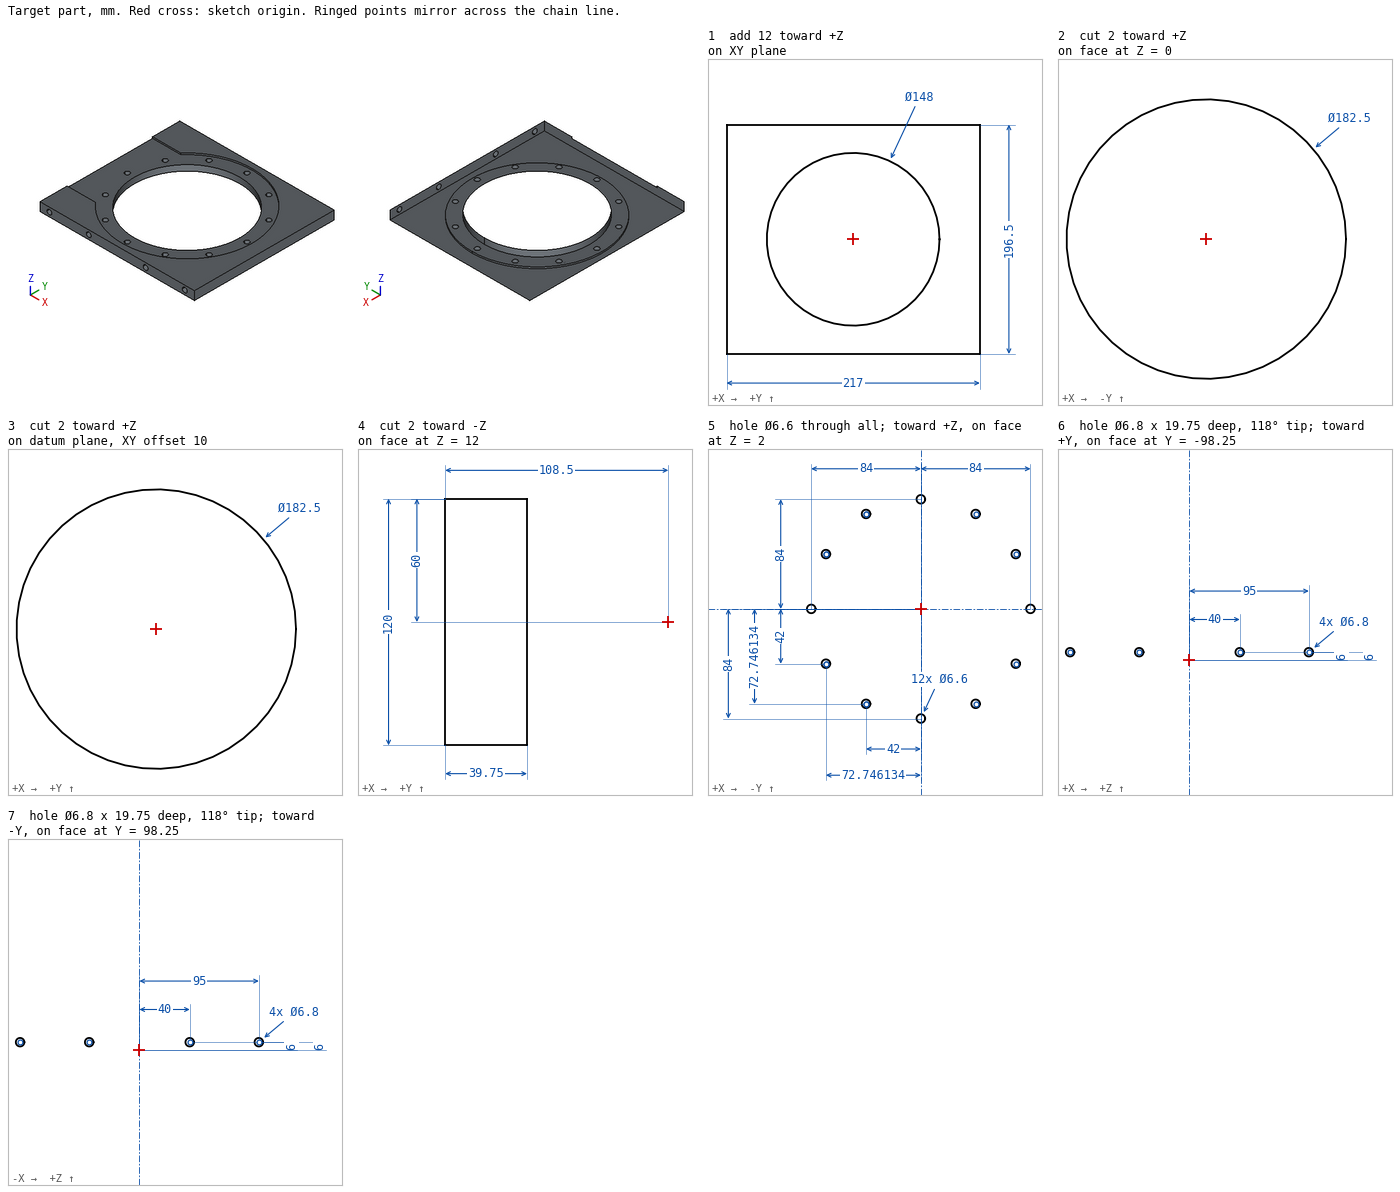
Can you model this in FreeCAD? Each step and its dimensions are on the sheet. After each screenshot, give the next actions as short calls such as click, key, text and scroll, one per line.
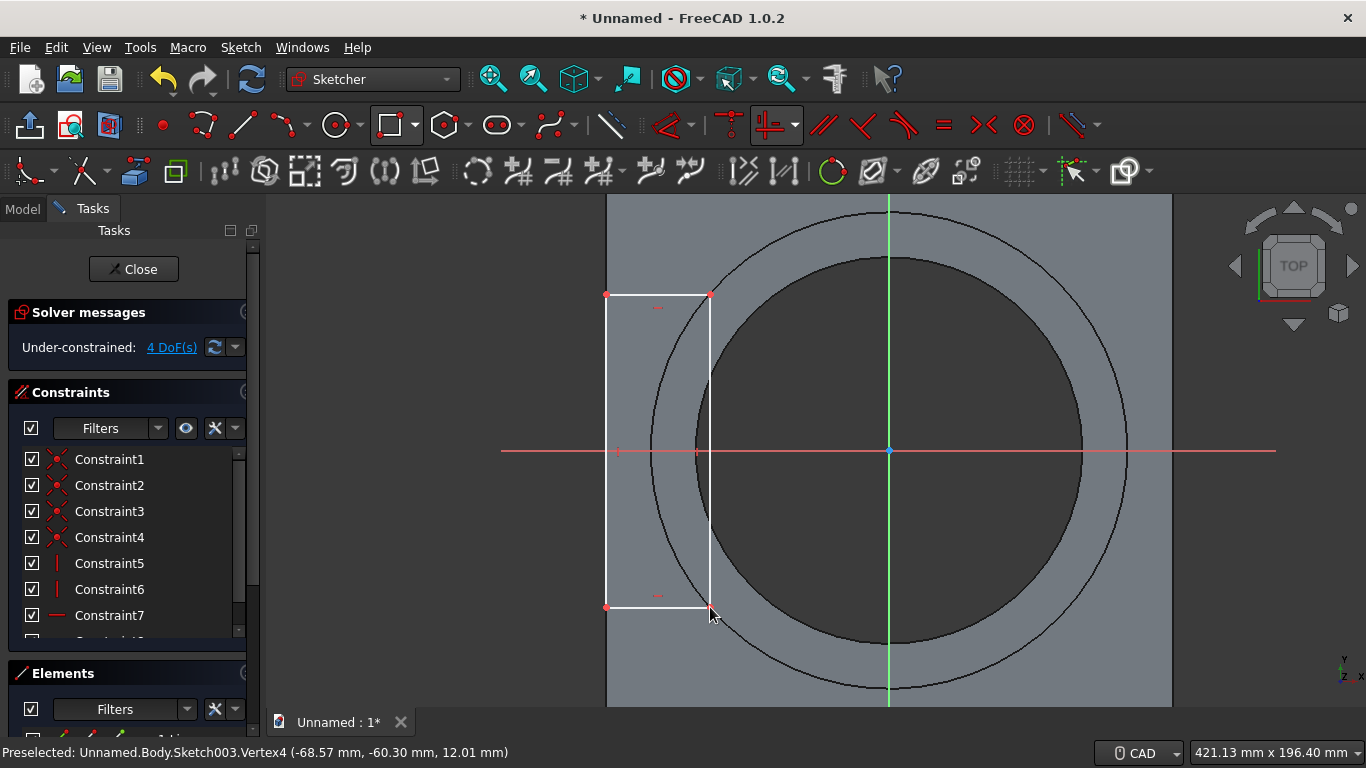
click(666, 126)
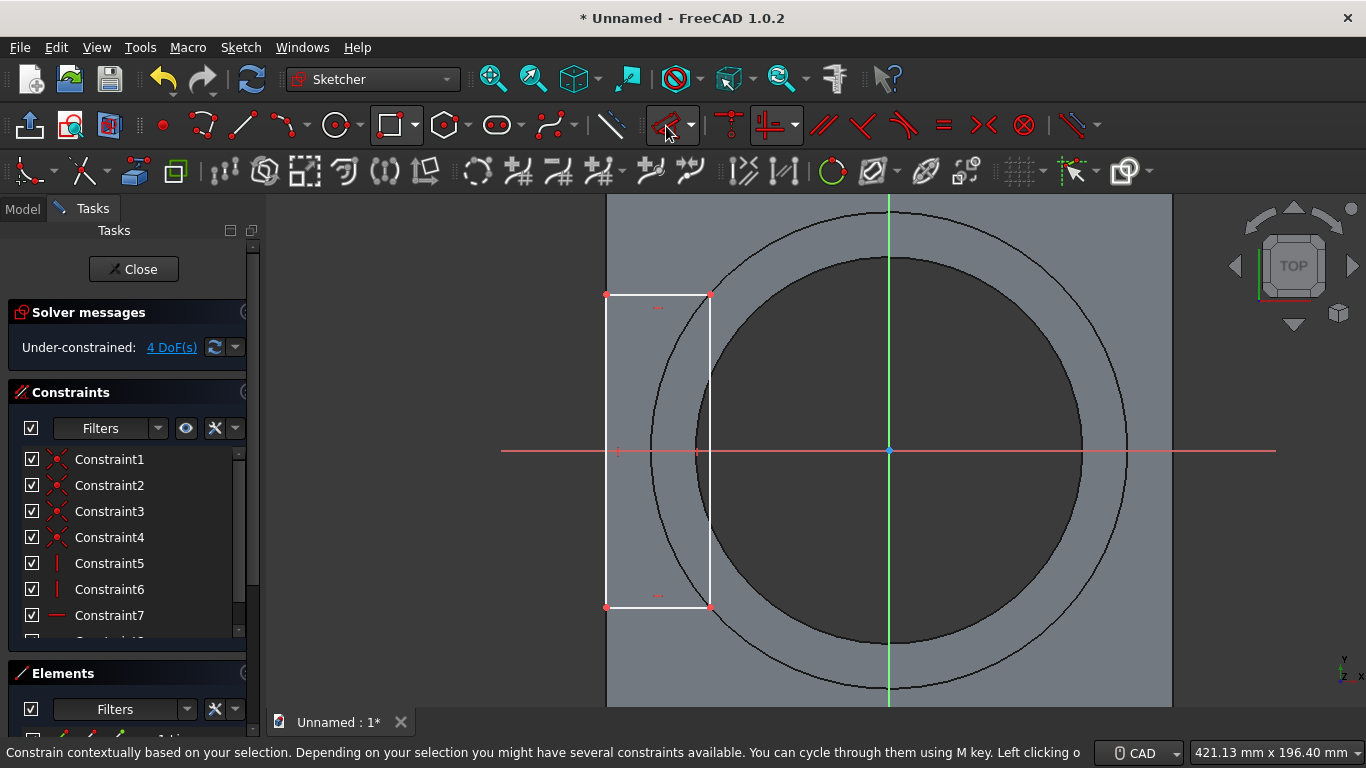
click(606, 389)
click(572, 380)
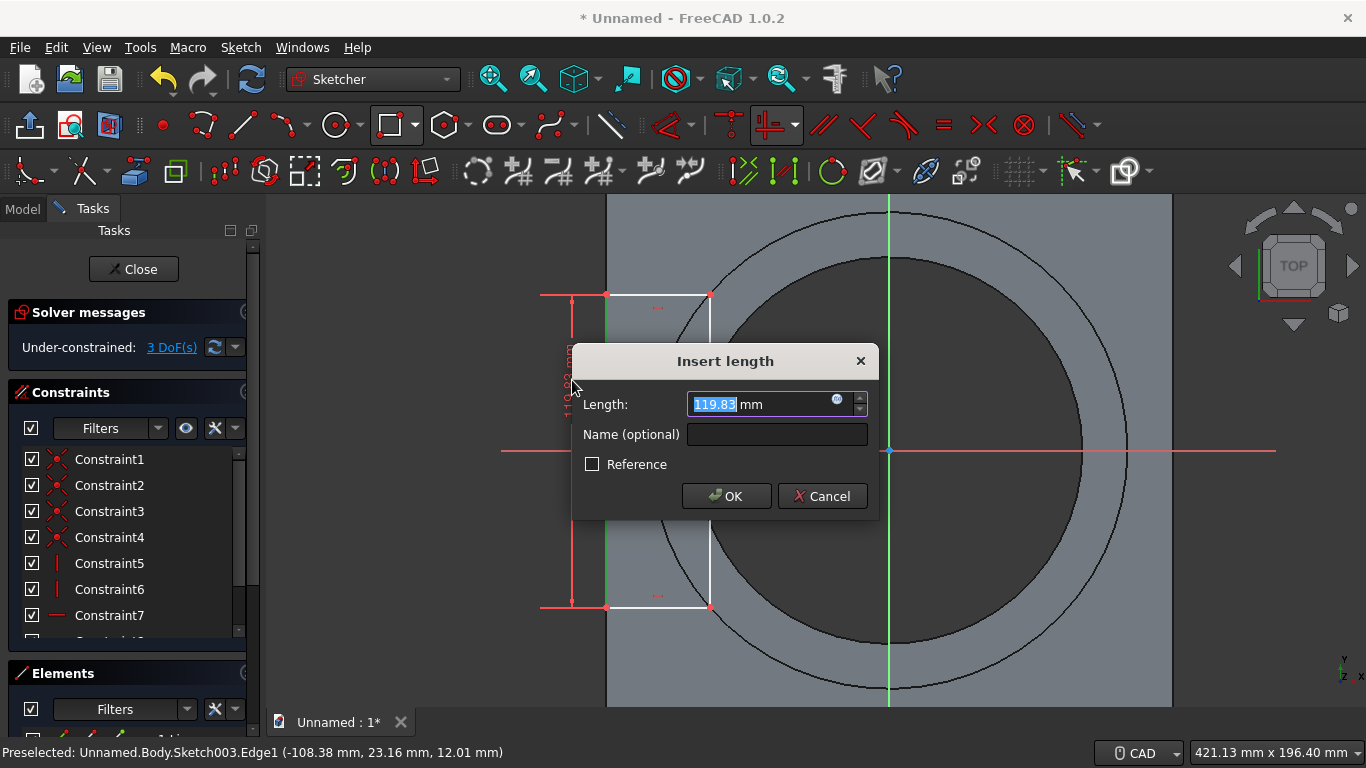
text(120)
key(Return)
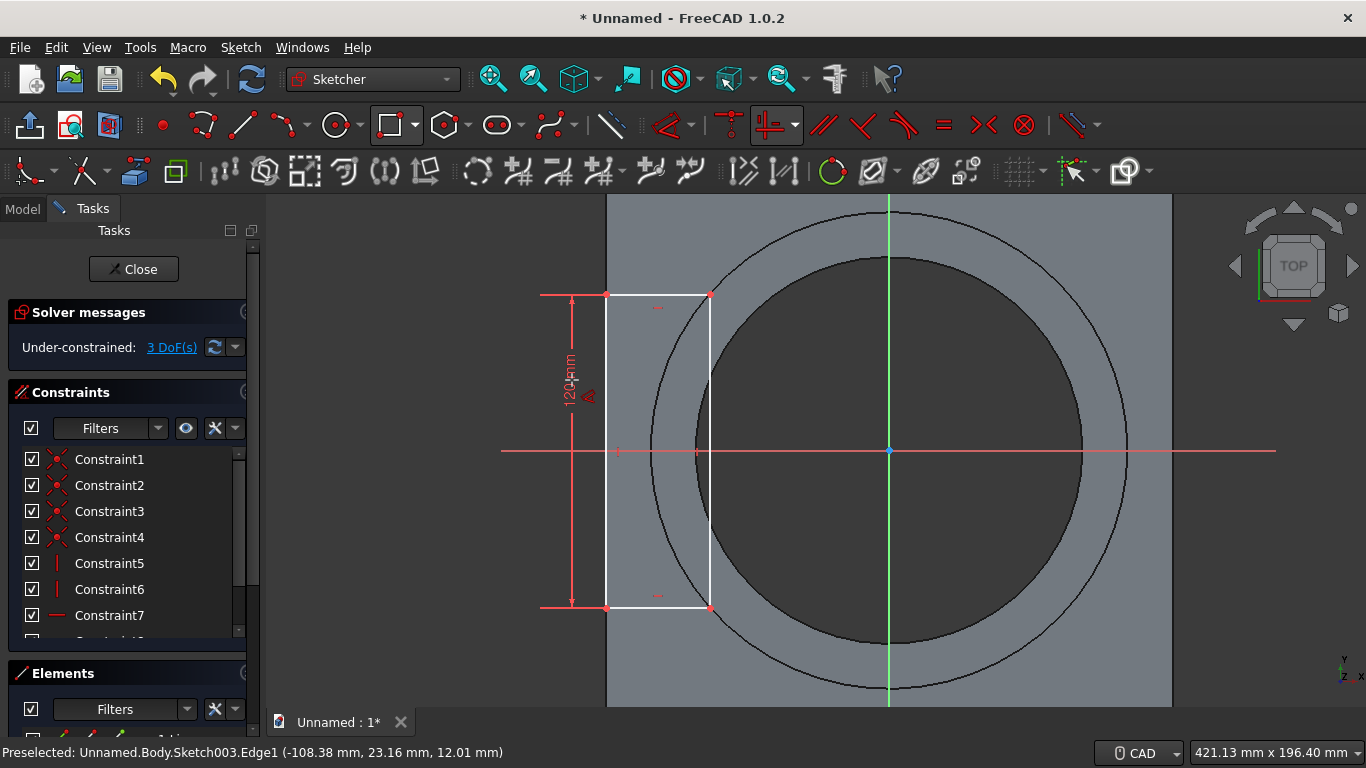
click(606, 295)
click(923, 373)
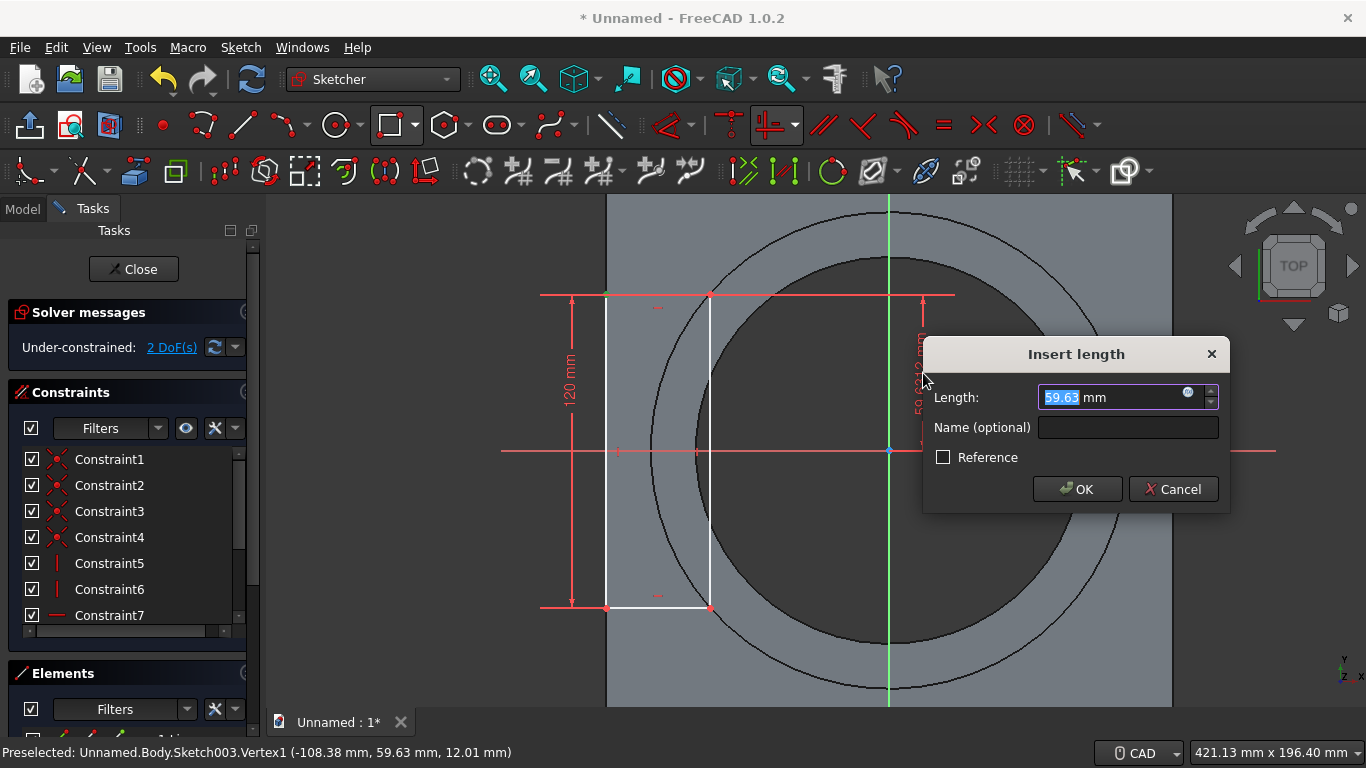
text(60)
key(Return)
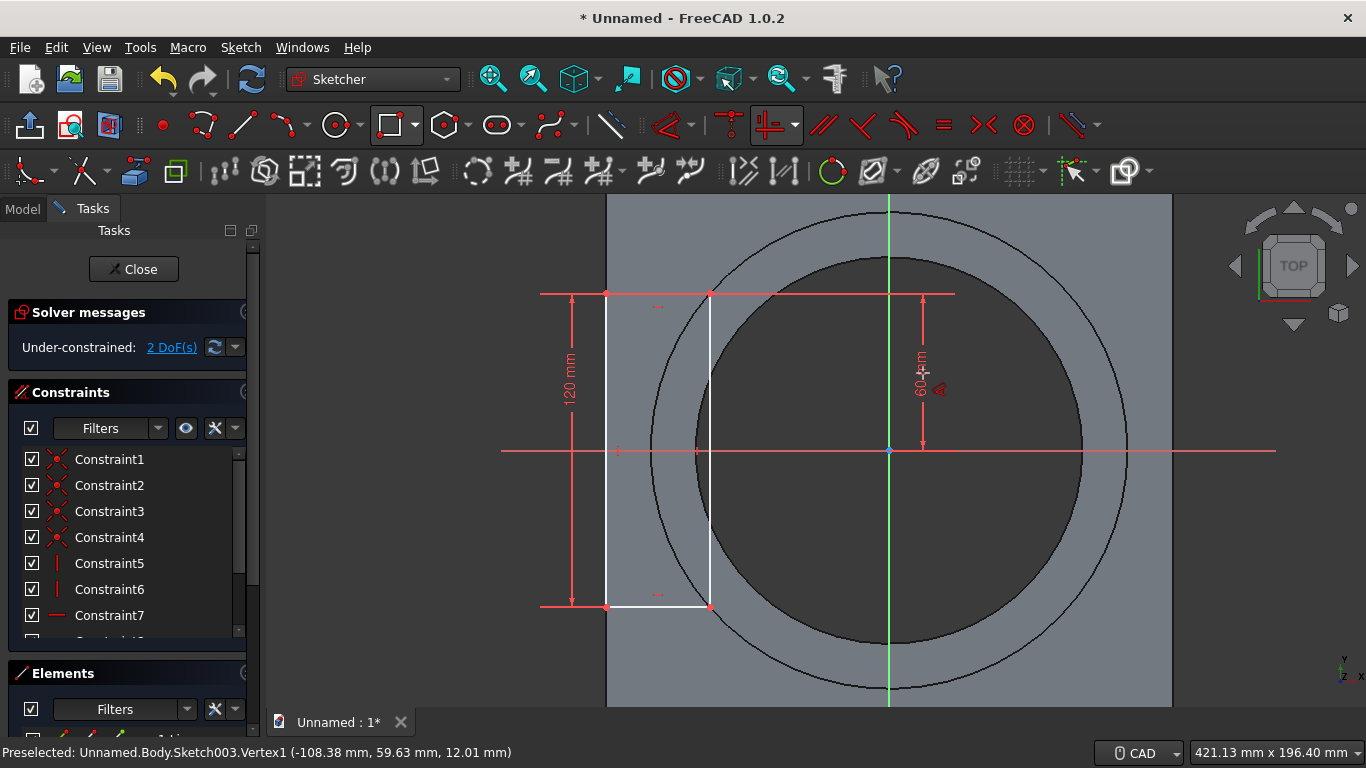
click(637, 607)
click(658, 641)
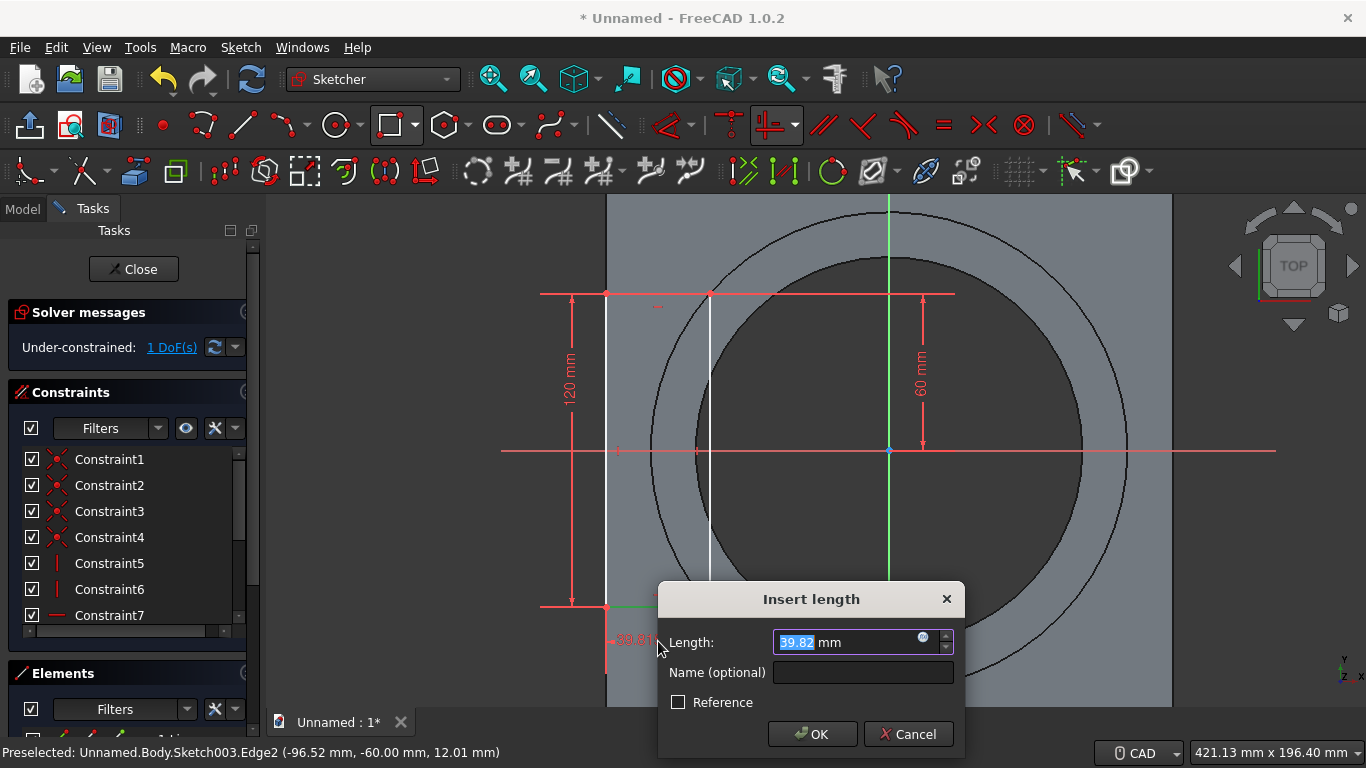
text(39.75)
key(Return)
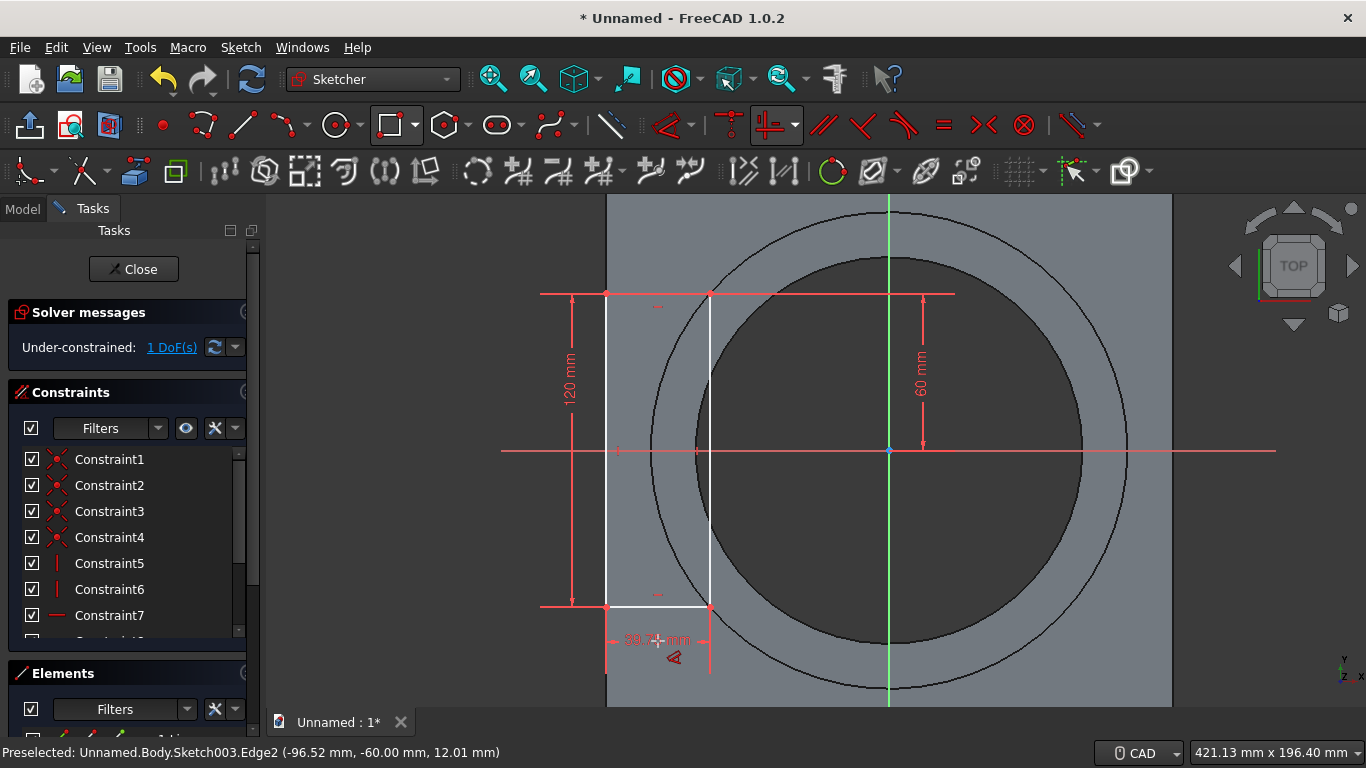
click(606, 294)
click(748, 260)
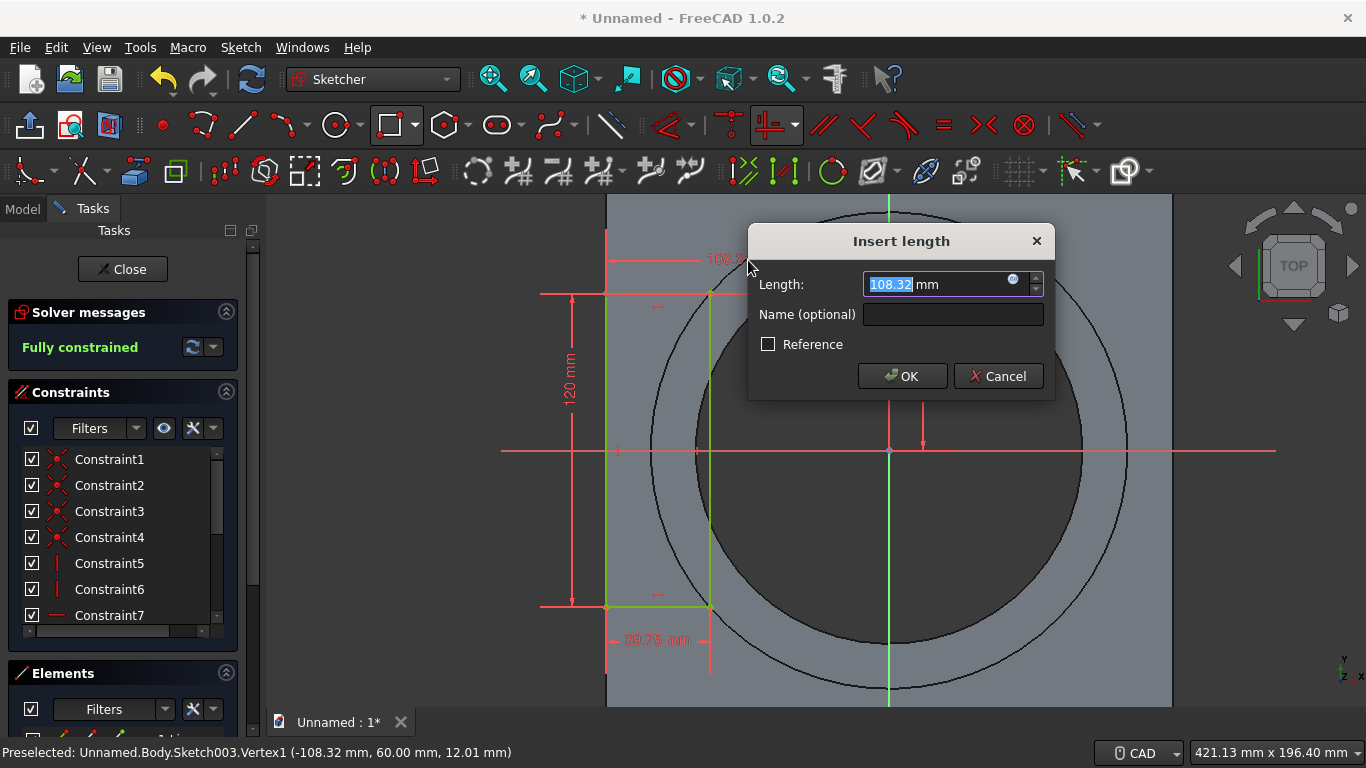
text(108.5)
key(Return)
key(Escape)